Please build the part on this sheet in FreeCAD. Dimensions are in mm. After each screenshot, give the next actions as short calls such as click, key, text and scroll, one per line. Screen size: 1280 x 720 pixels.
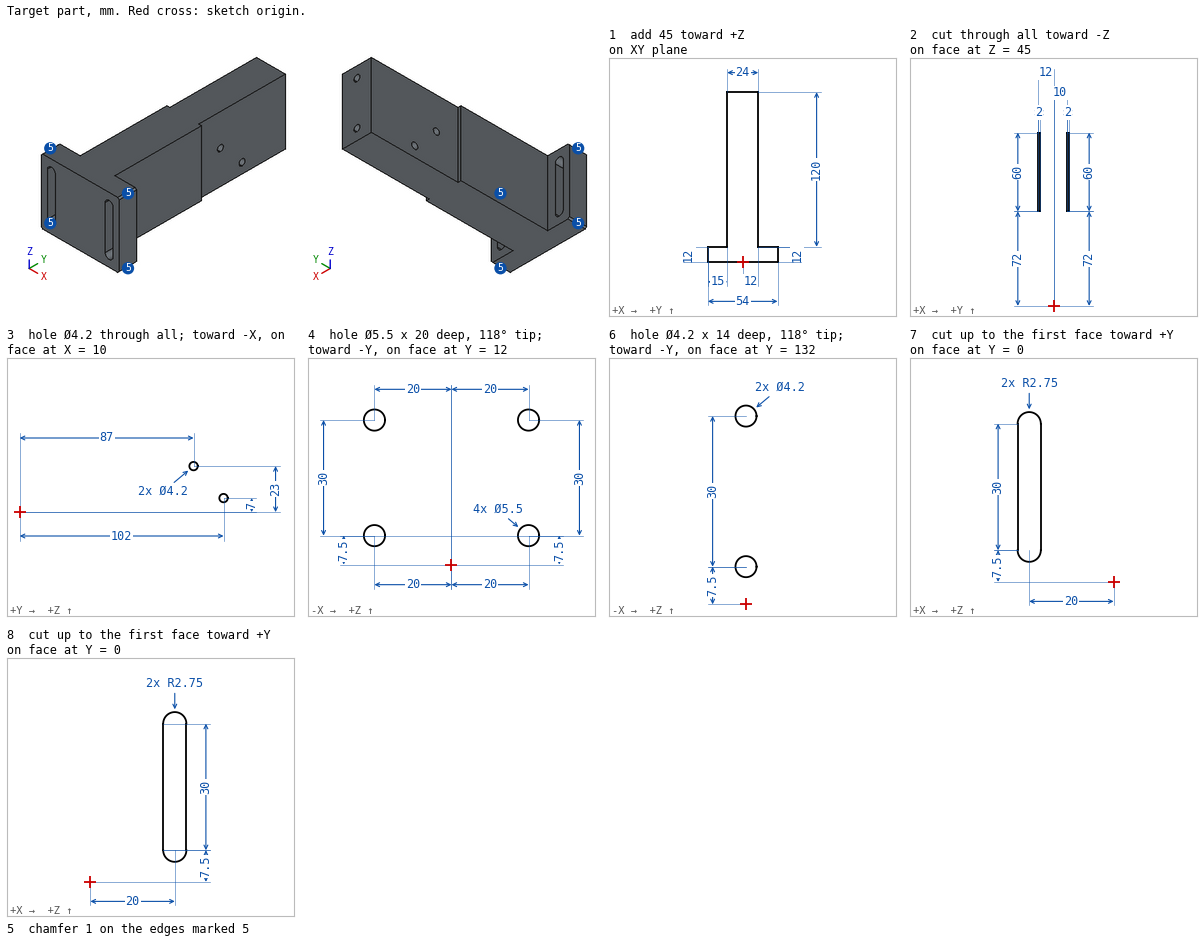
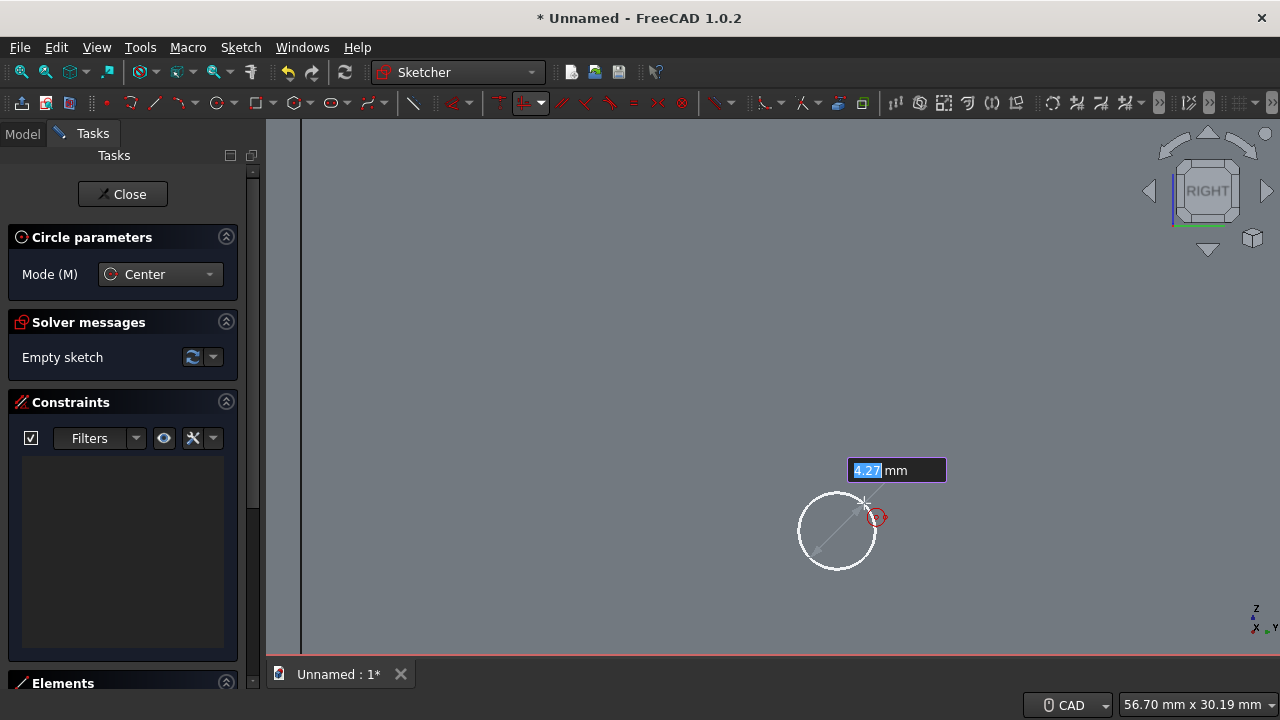
text(4.2)
key(Return)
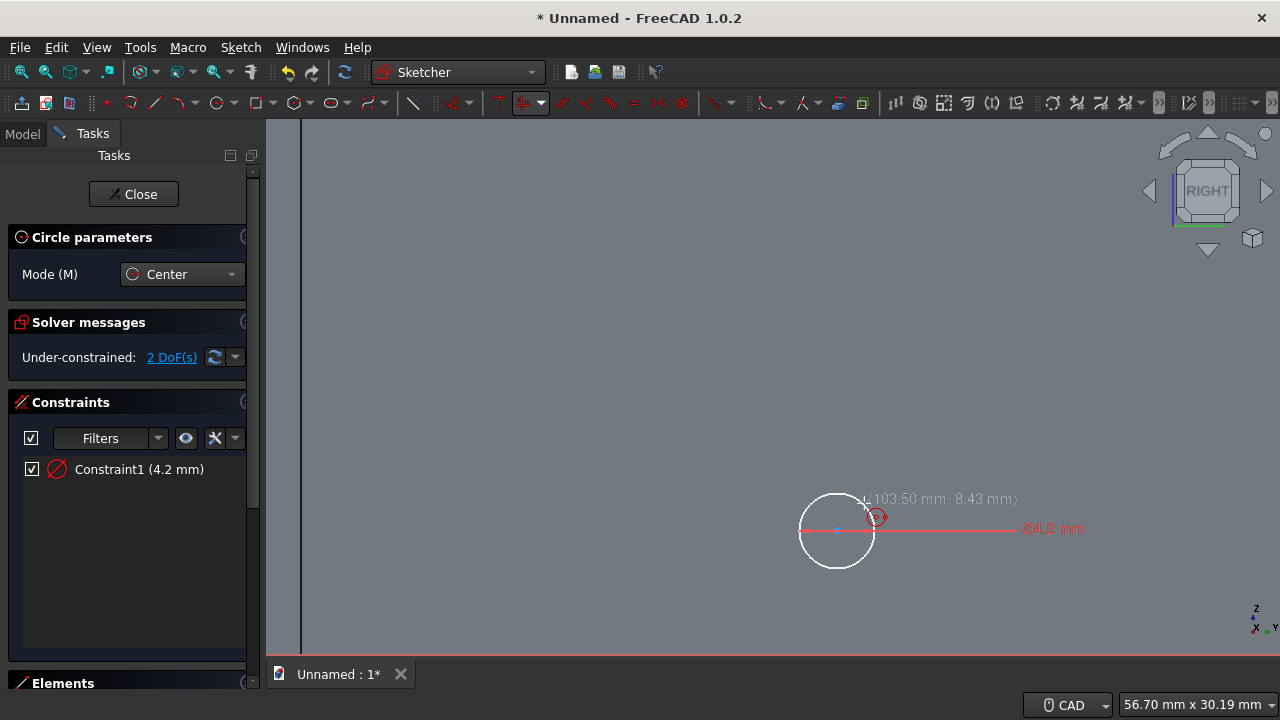
click(569, 243)
move(595, 217)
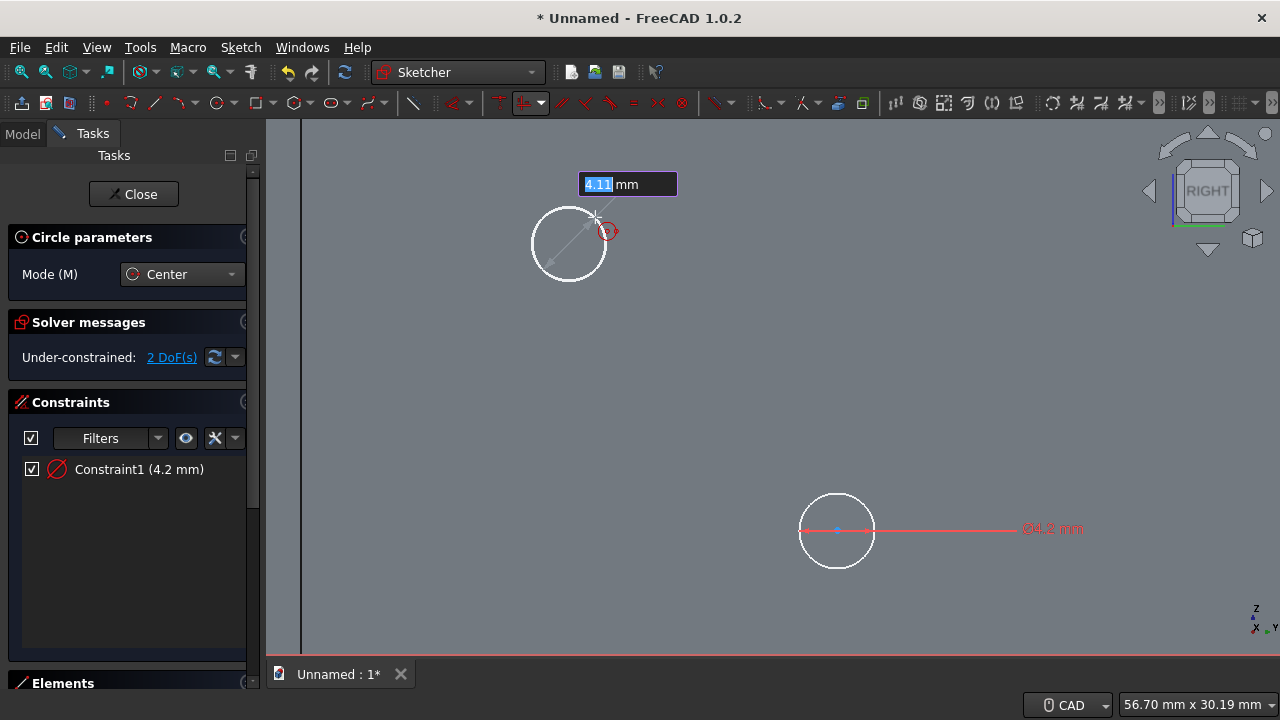
text(4.2)
key(Return)
key(Escape)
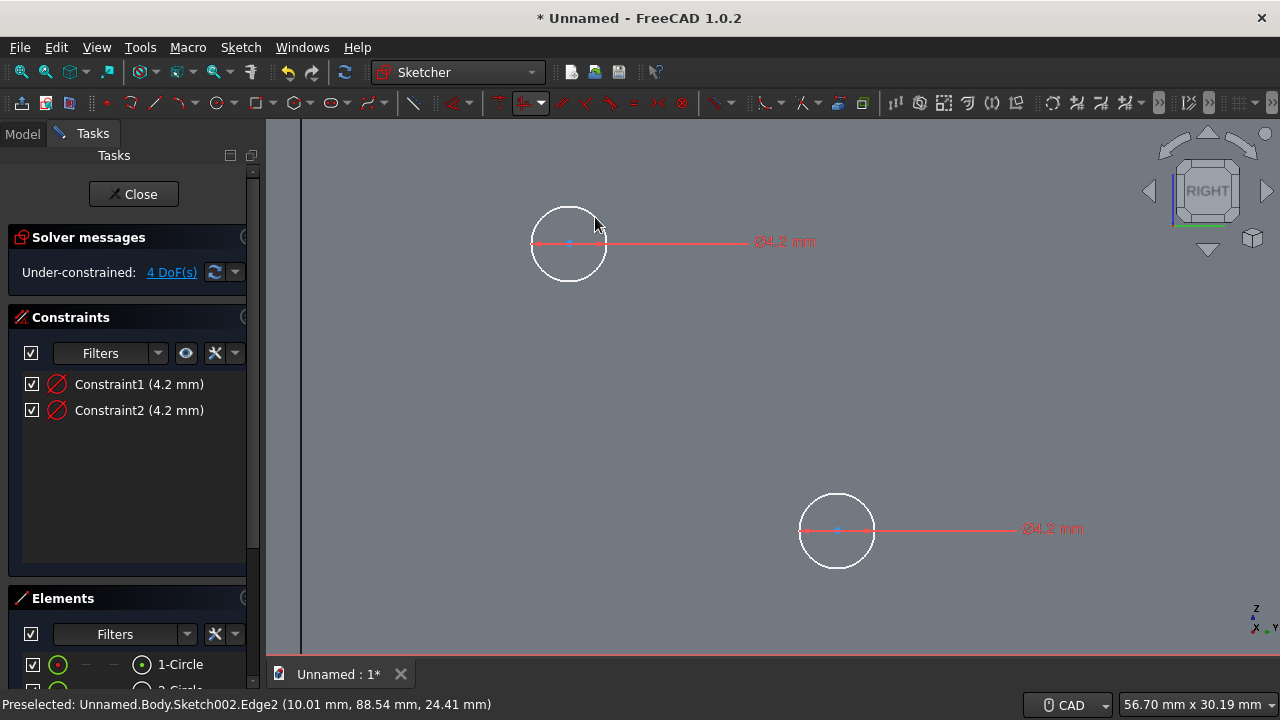
click(452, 104)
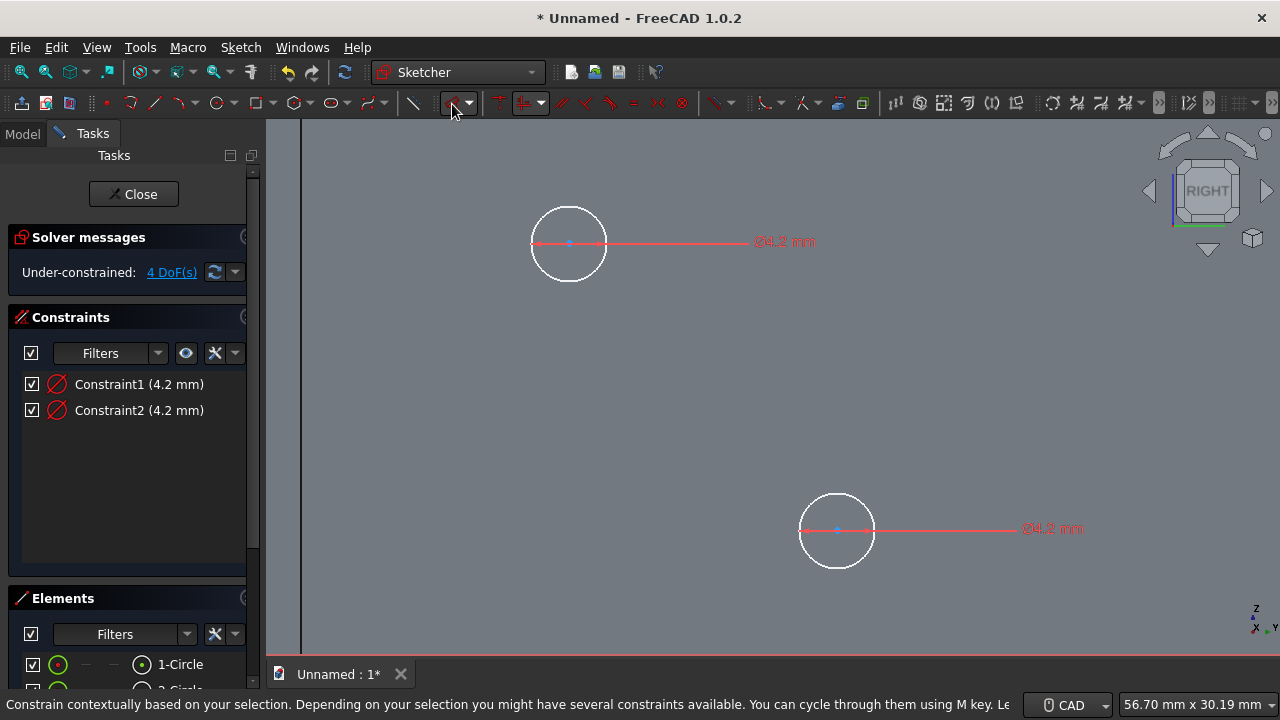
click(837, 531)
click(871, 581)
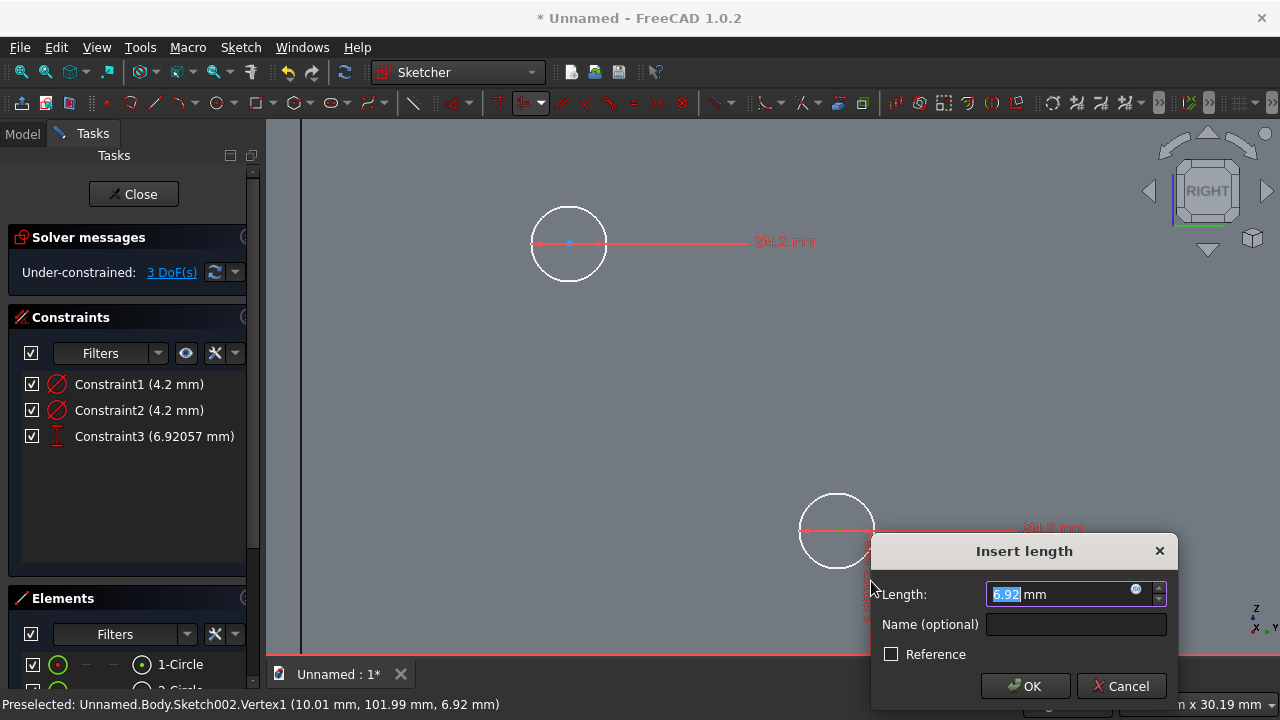
text(7)
key(Return)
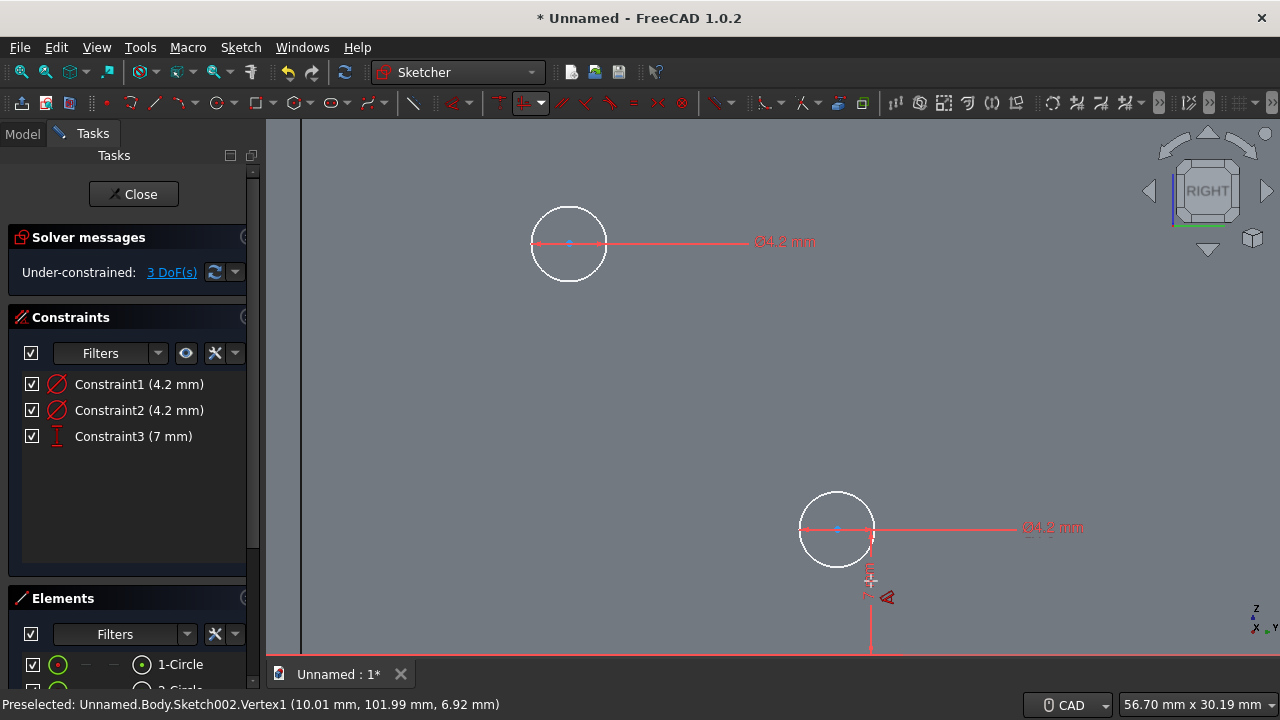
click(569, 244)
click(431, 210)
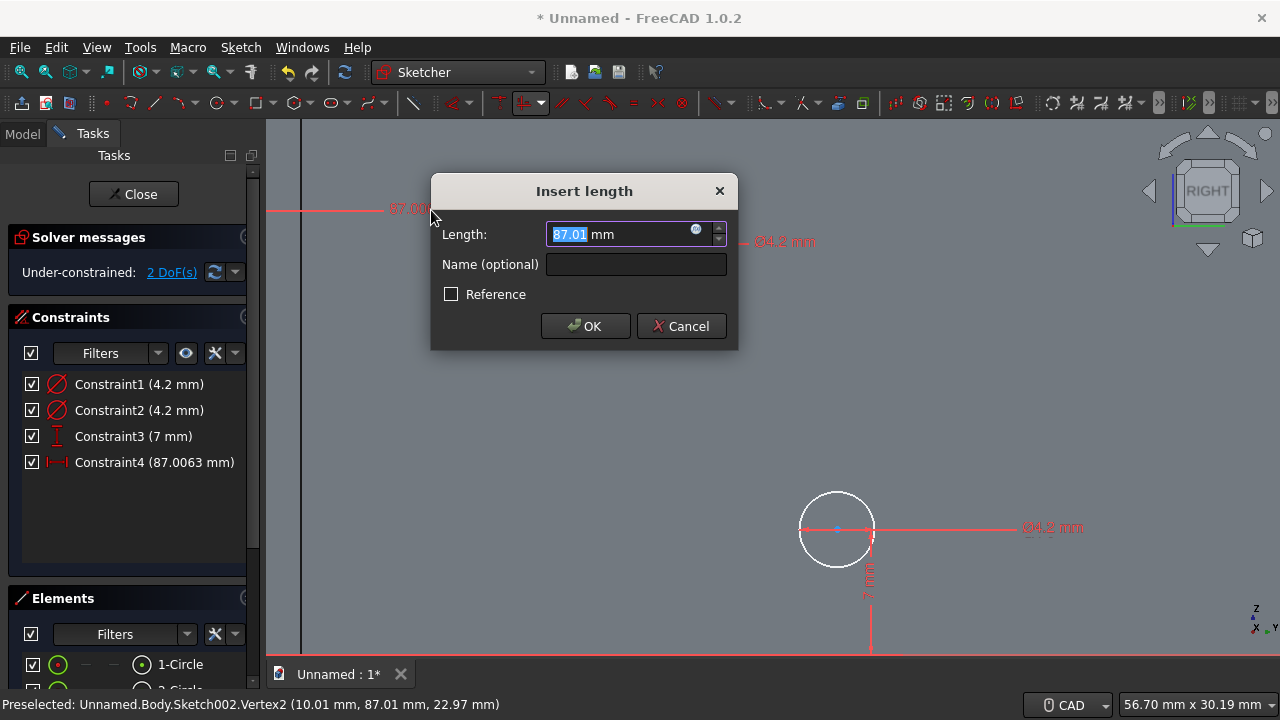
text(87)
key(Return)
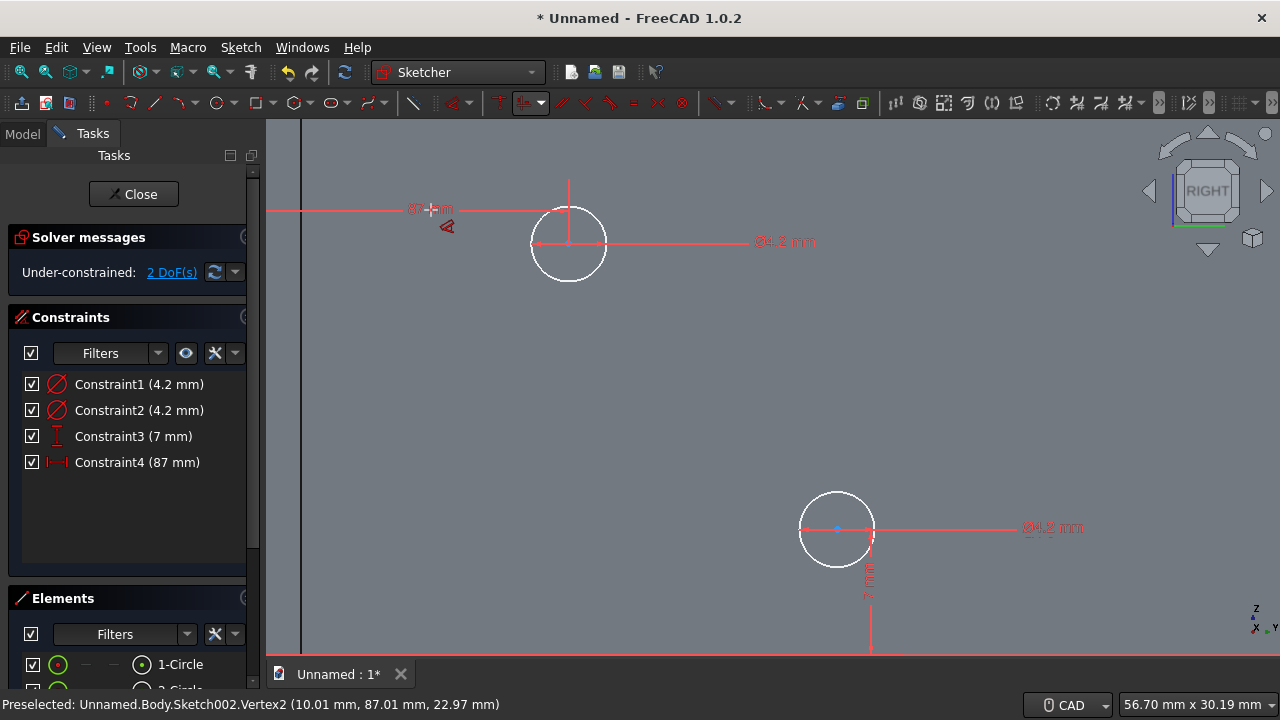
click(569, 244)
click(603, 438)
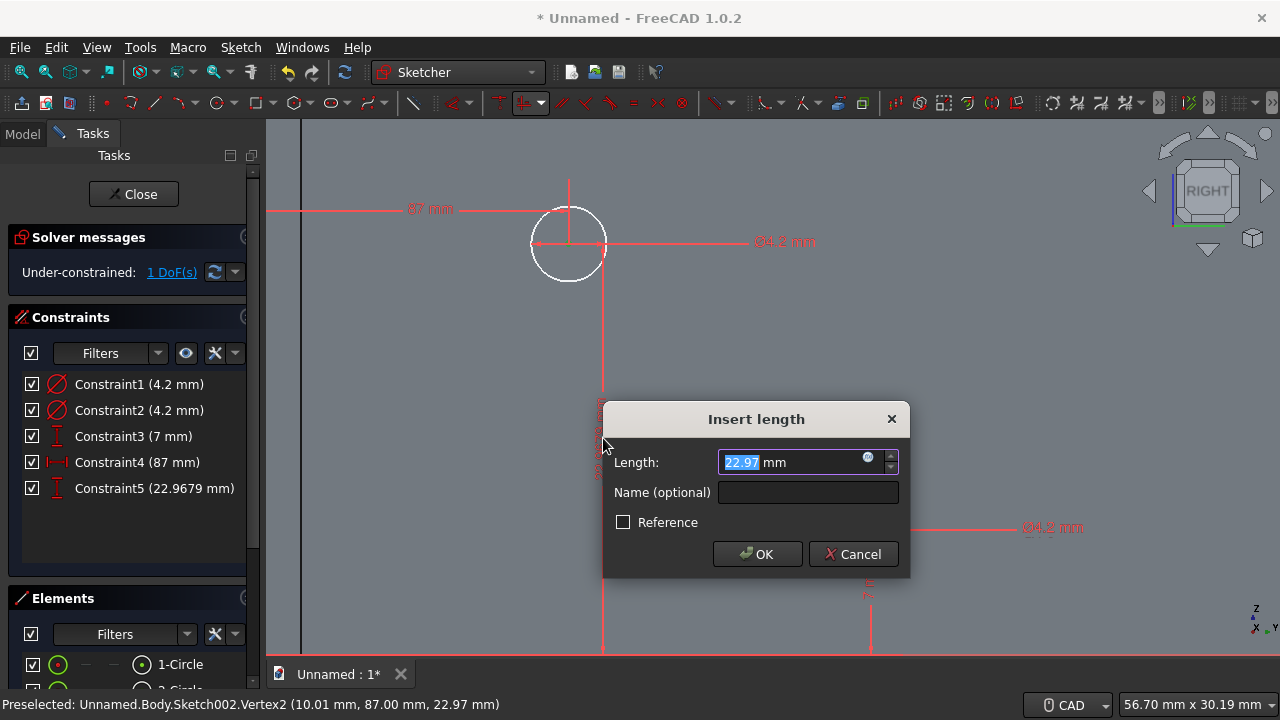
text(23)
key(Return)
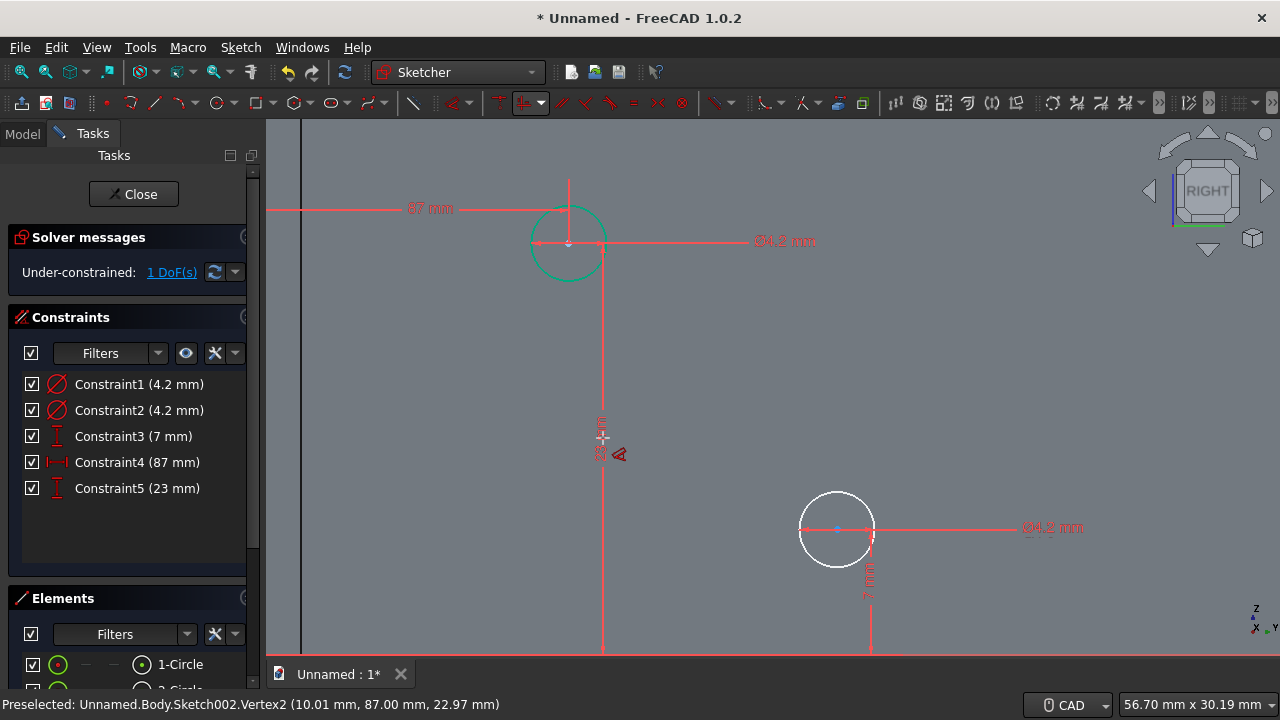
click(837, 530)
click(566, 496)